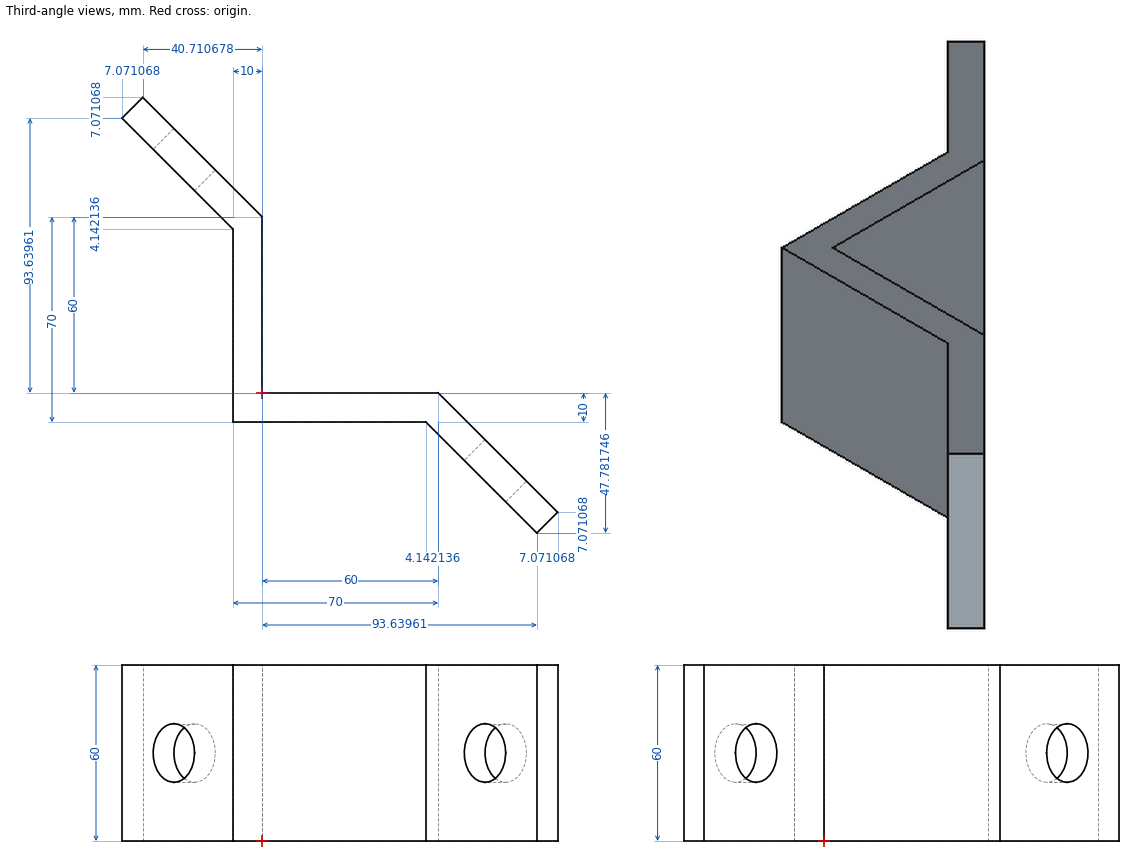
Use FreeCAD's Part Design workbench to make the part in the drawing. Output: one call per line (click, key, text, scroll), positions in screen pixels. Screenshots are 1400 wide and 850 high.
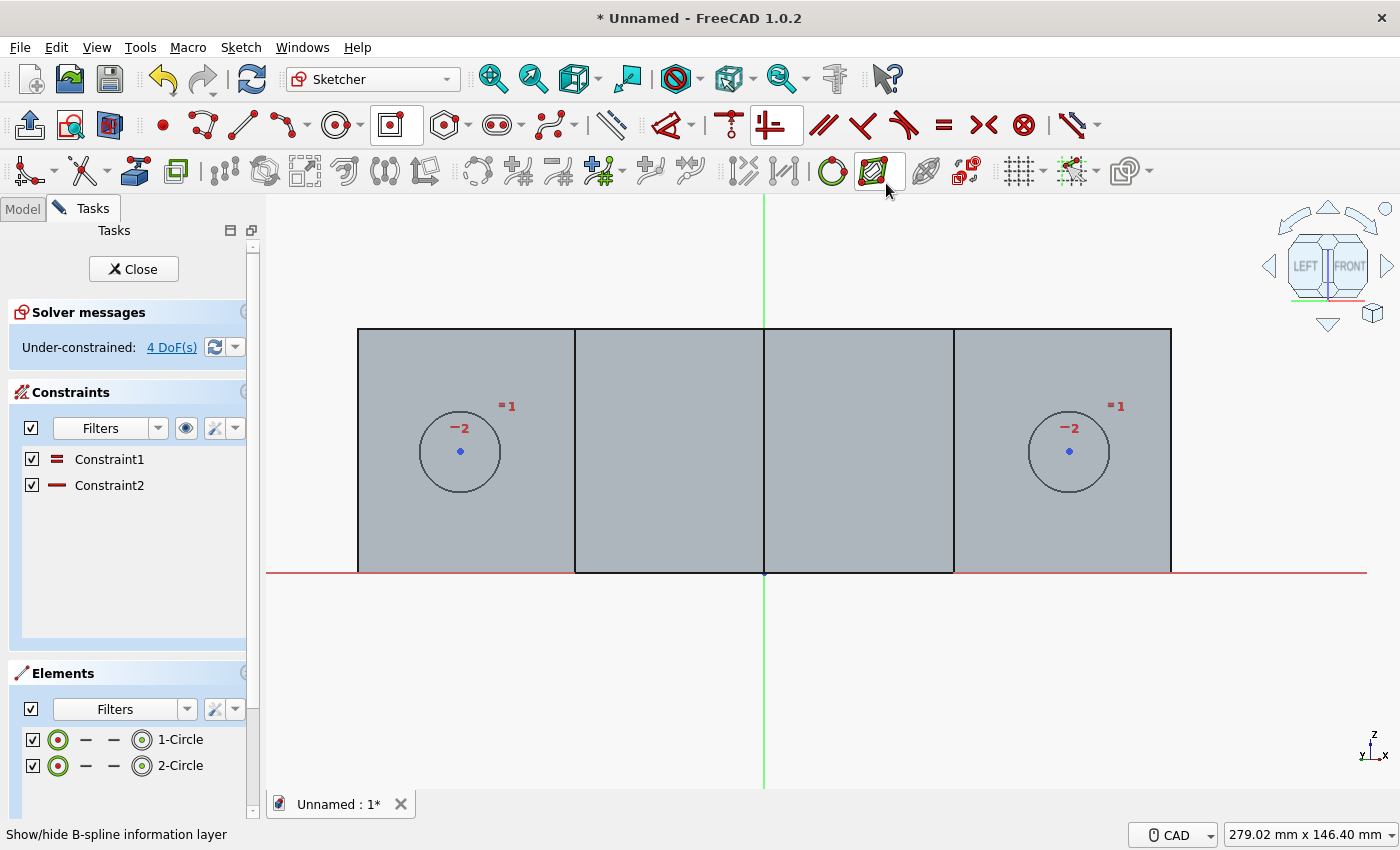
click(666, 126)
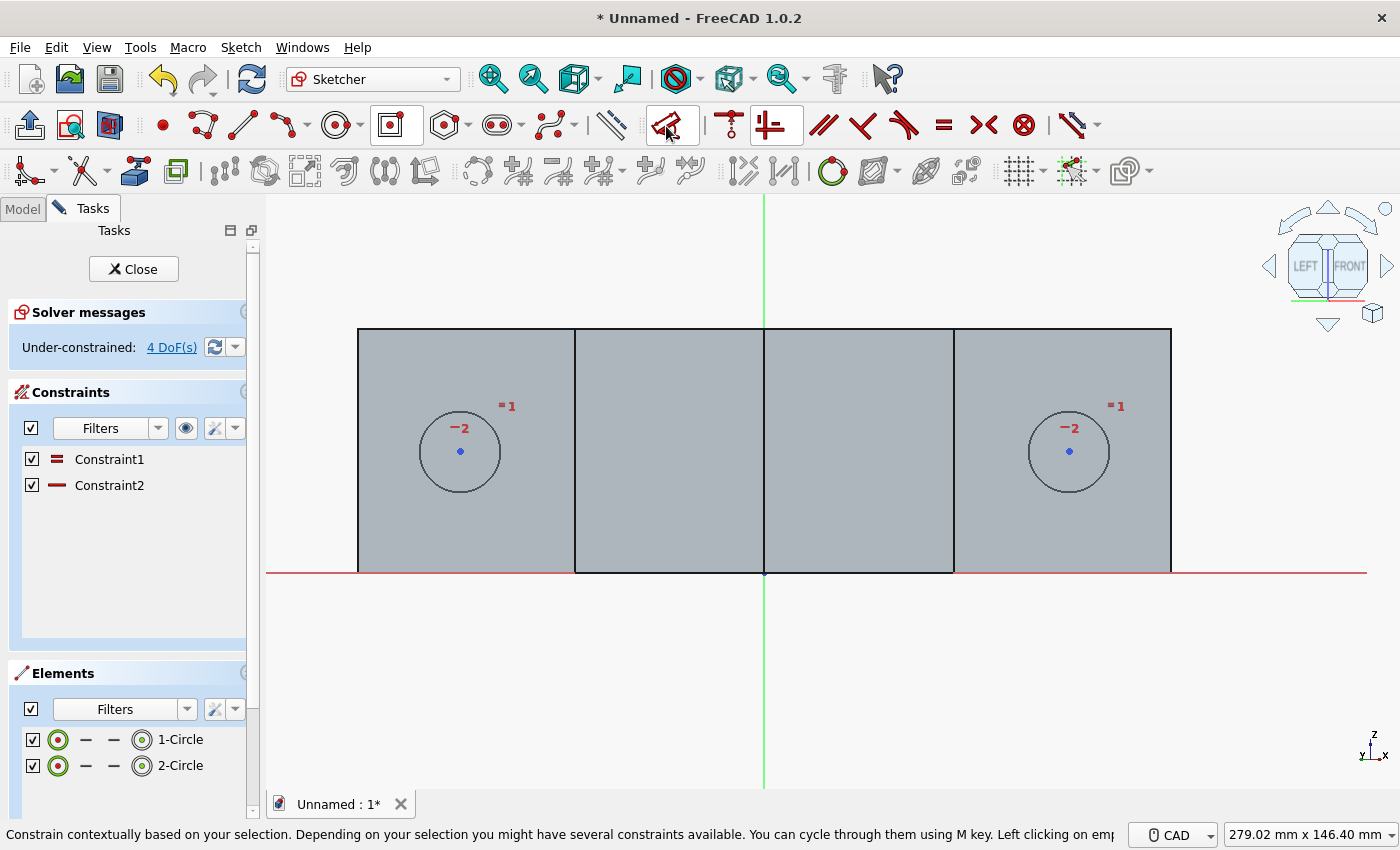
click(488, 423)
click(510, 400)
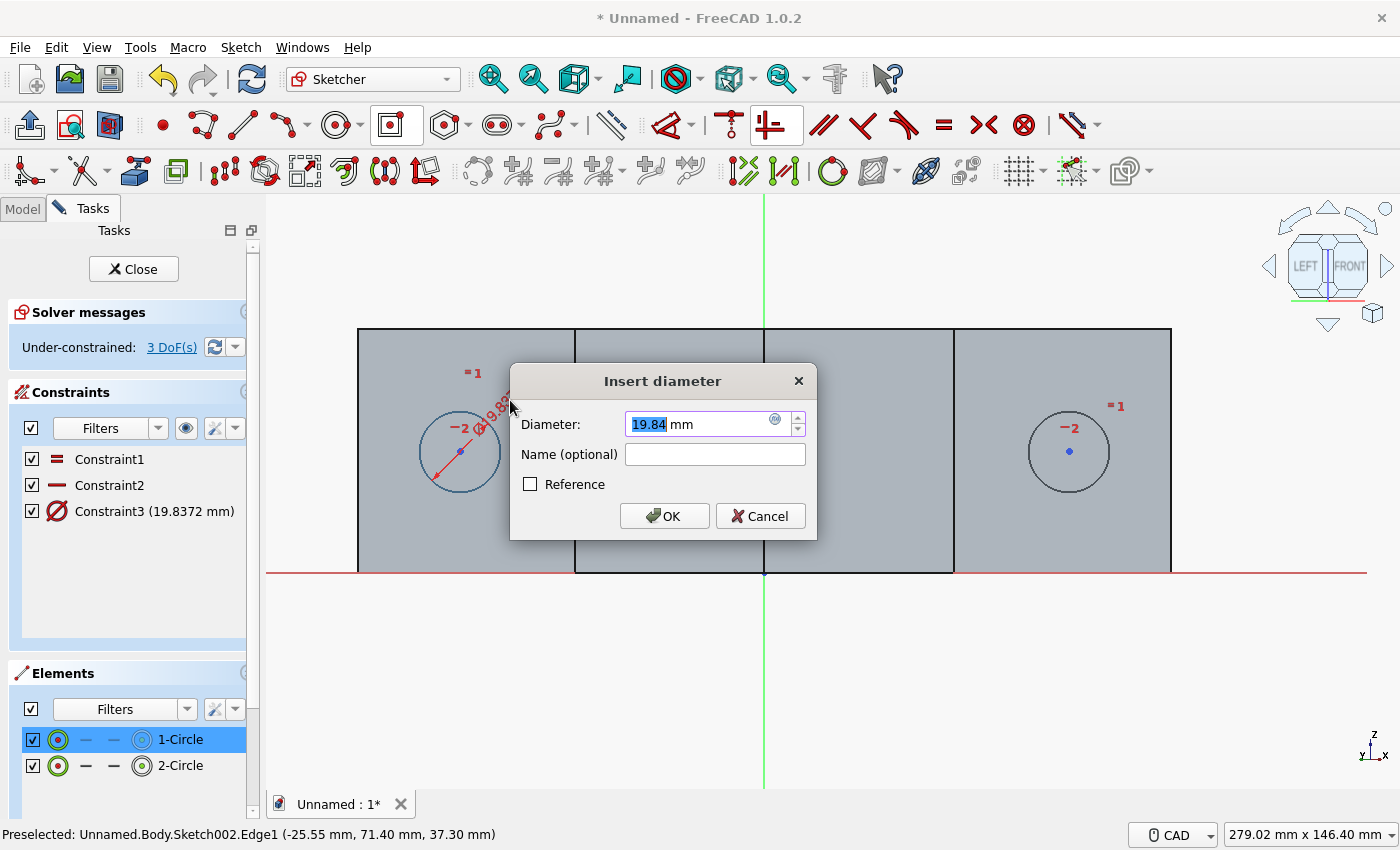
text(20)
key(Return)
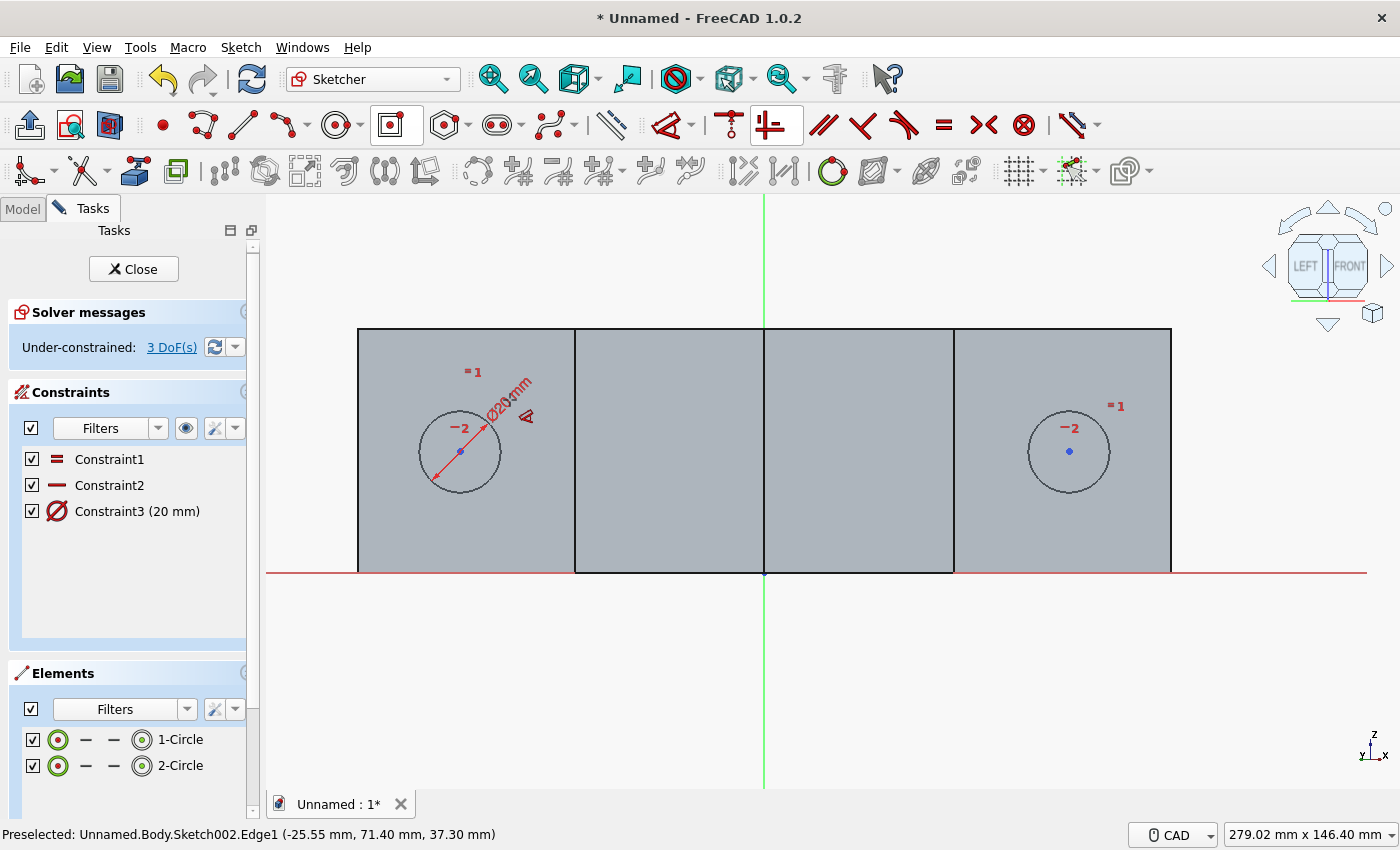
click(460, 452)
click(612, 607)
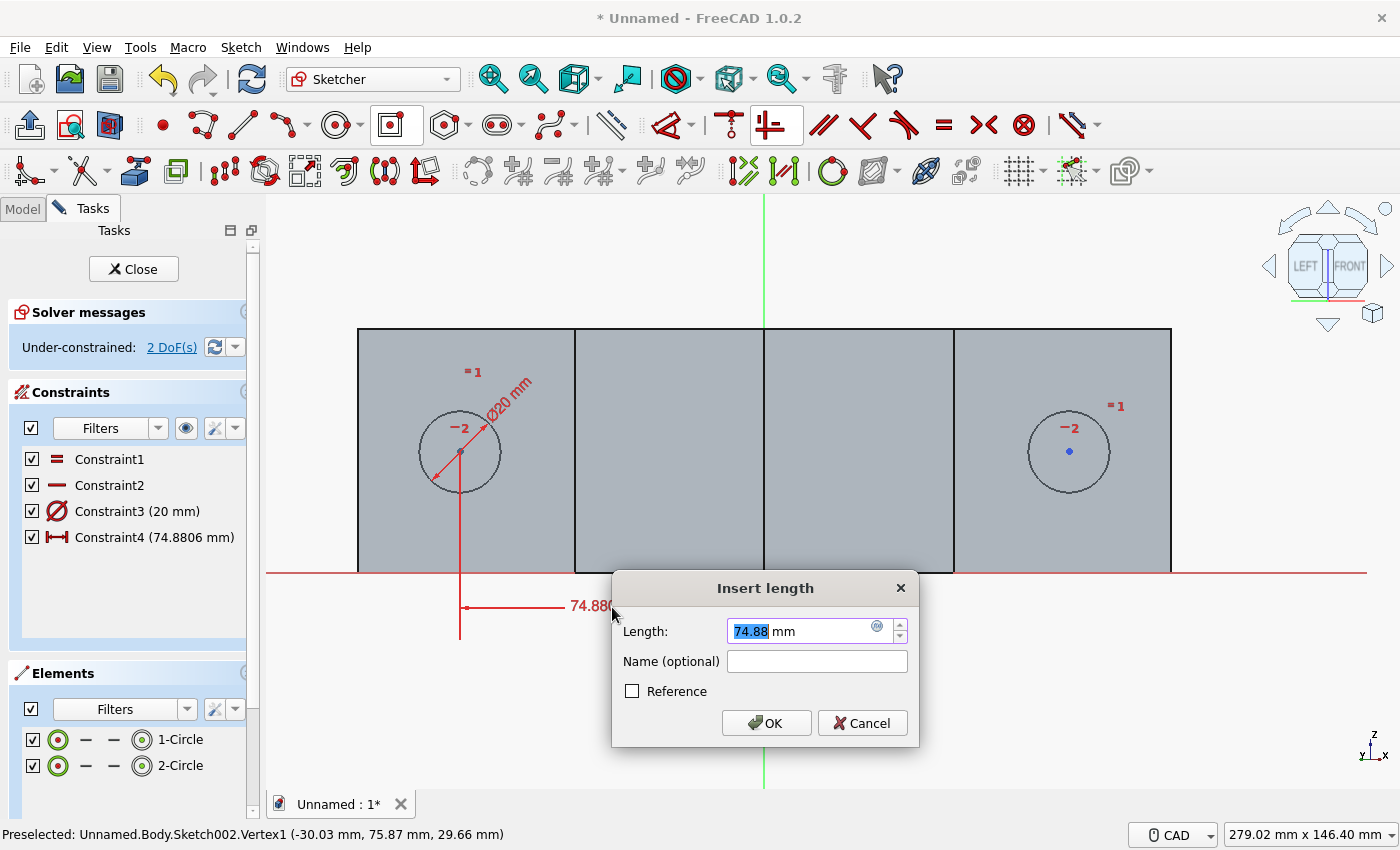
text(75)
key(Return)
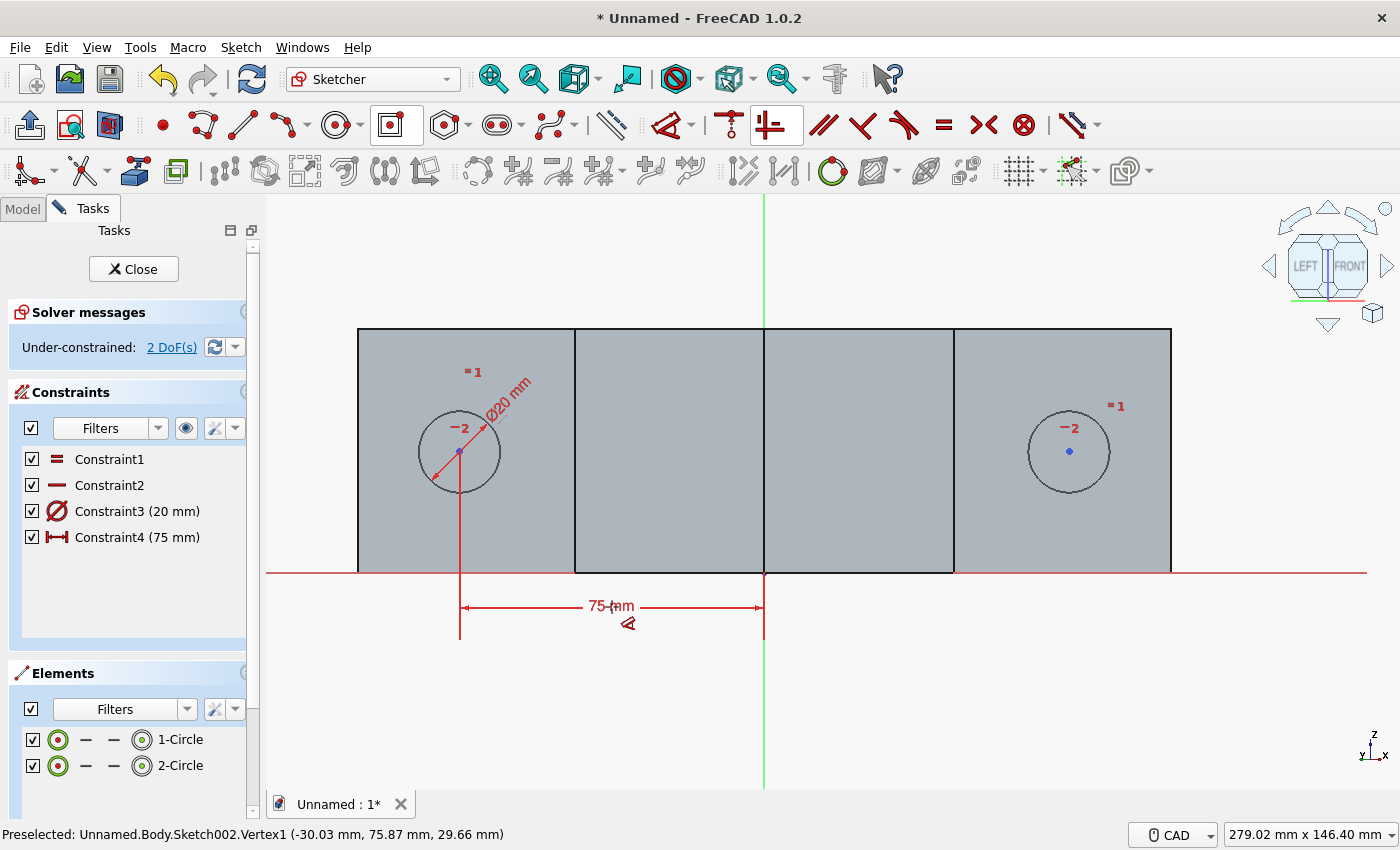
click(460, 452)
click(426, 512)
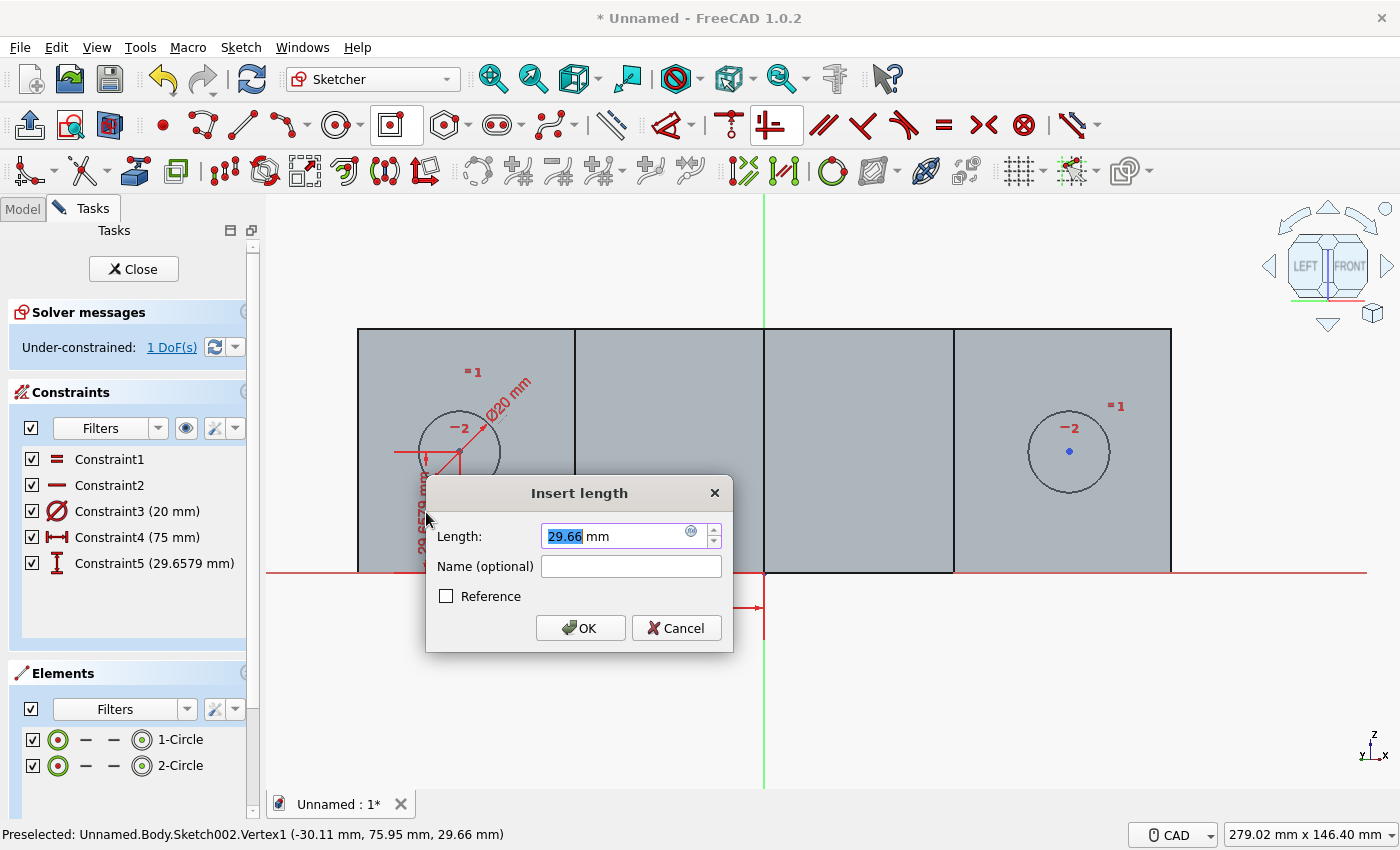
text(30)
key(Return)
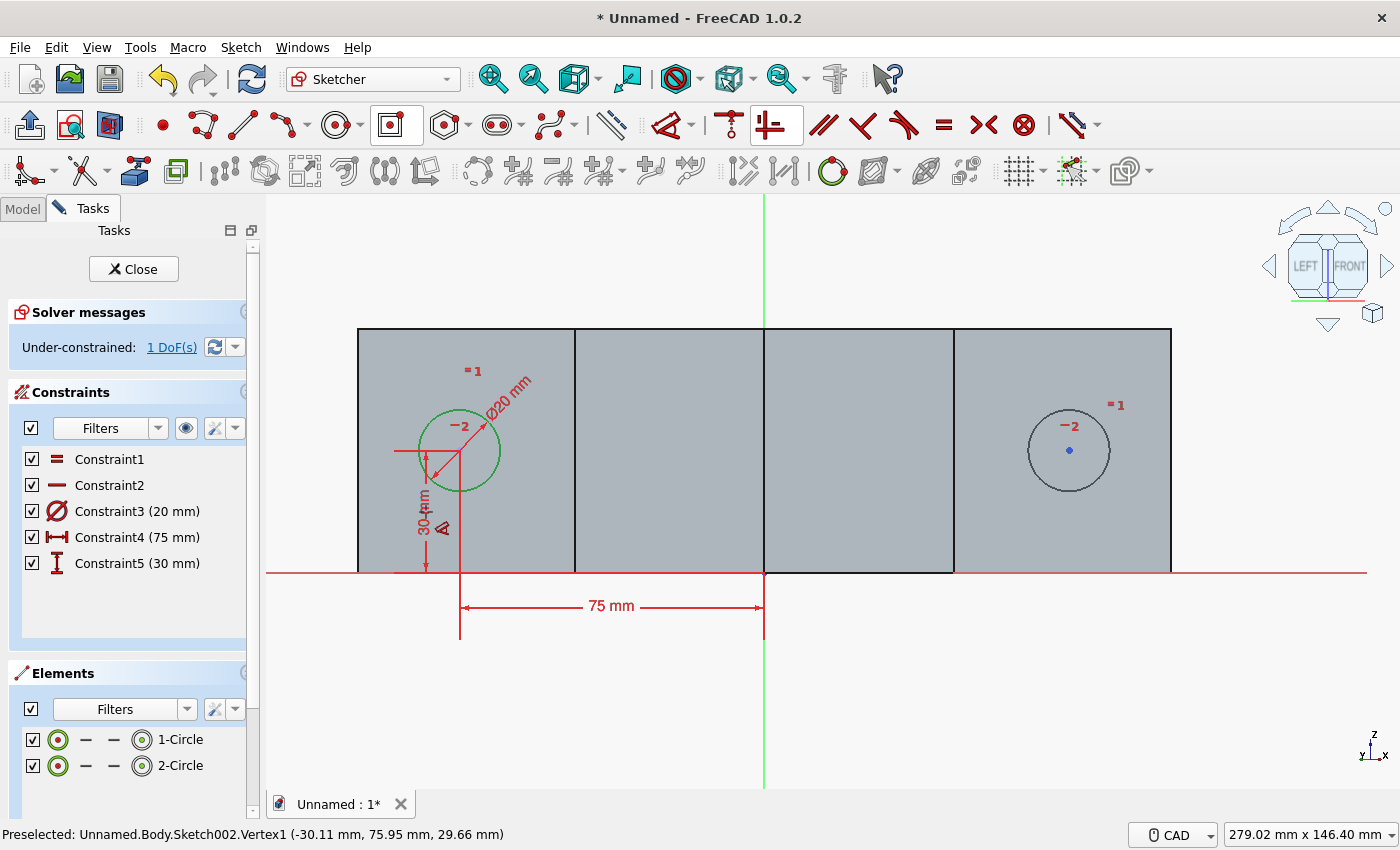
click(1069, 451)
click(917, 607)